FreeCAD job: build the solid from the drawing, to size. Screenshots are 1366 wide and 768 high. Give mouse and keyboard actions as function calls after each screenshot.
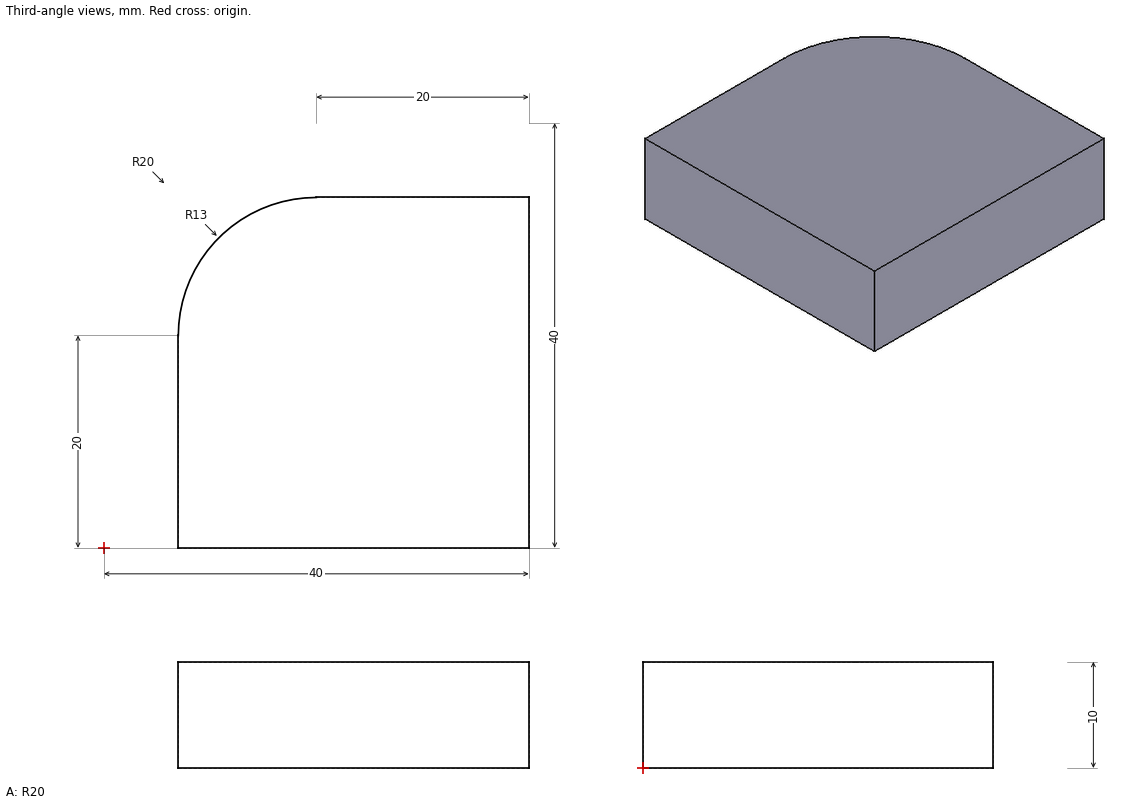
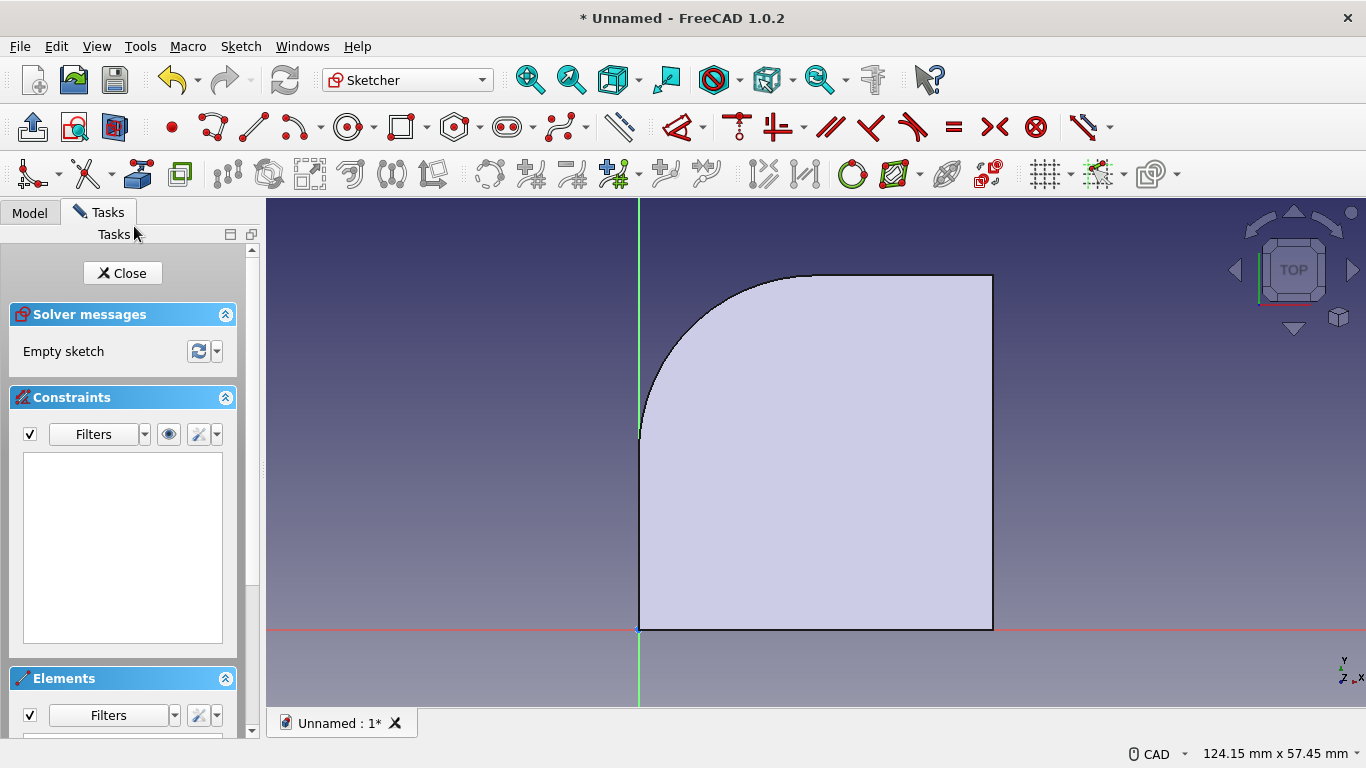
click(115, 128)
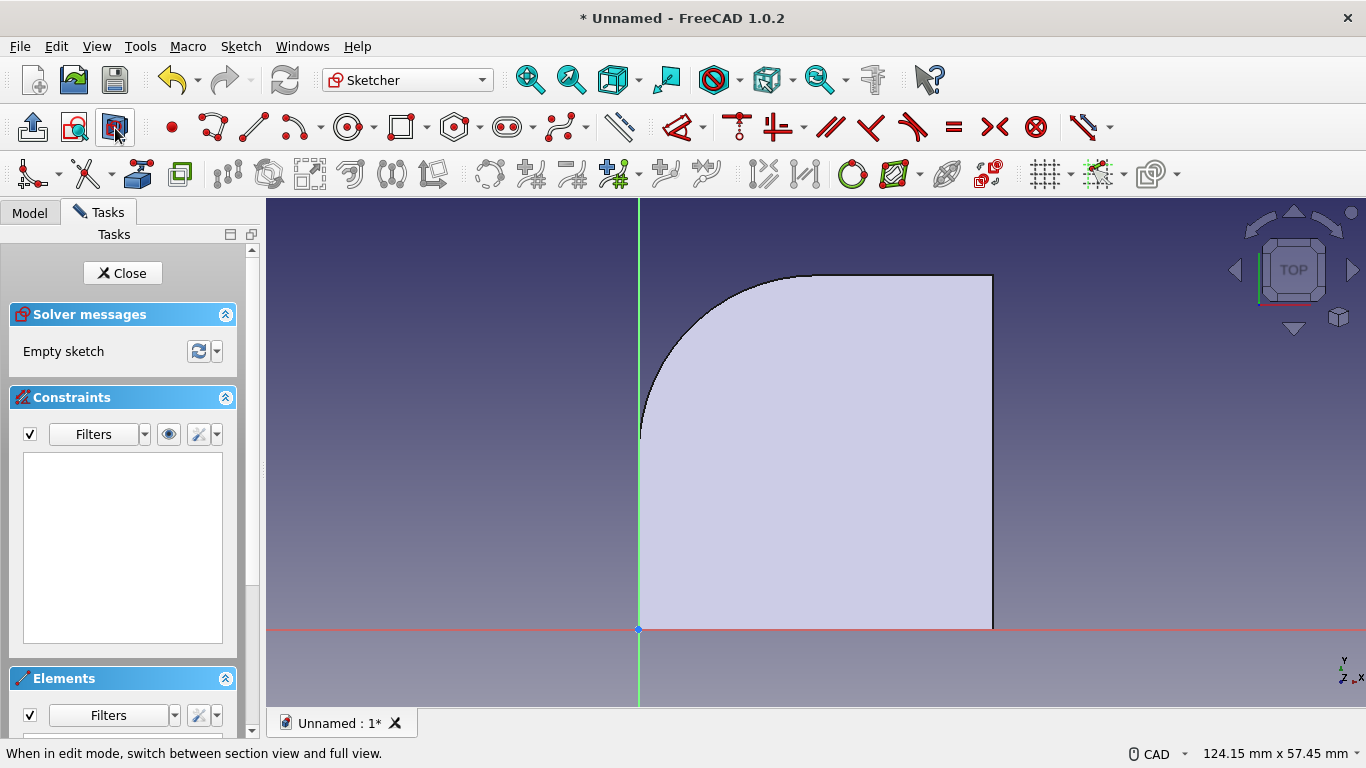
click(213, 128)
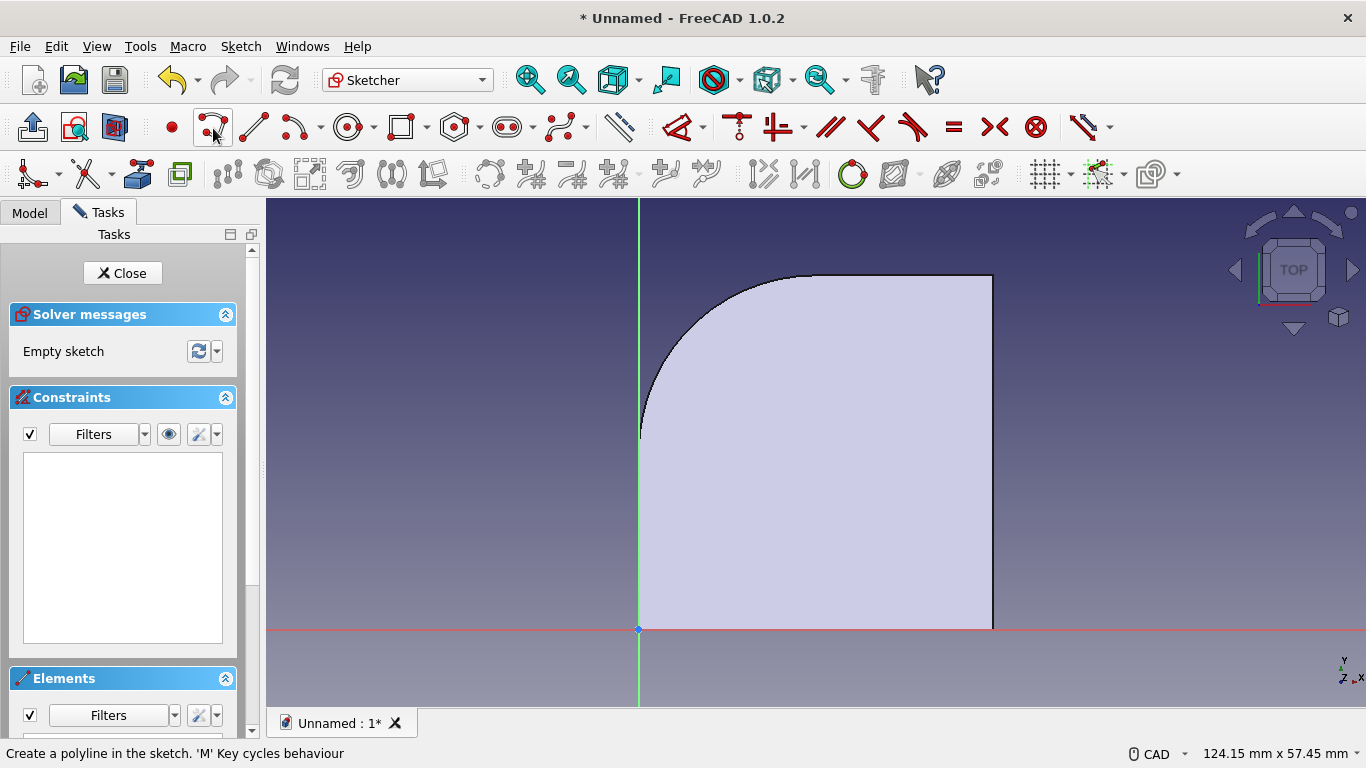
click(816, 275)
click(993, 275)
click(993, 337)
click(816, 337)
right_click(816, 337)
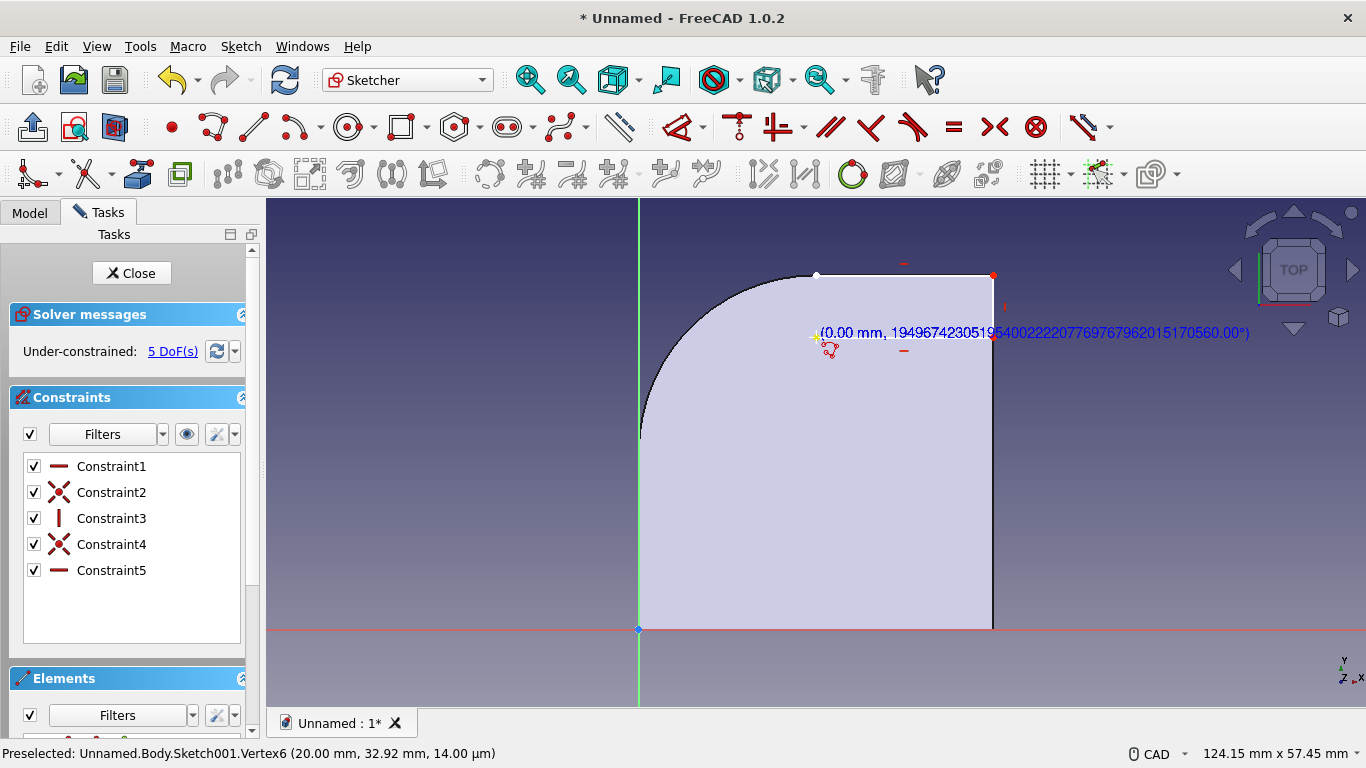
click(701, 452)
click(701, 630)
click(639, 630)
click(648, 452)
right_click(648, 452)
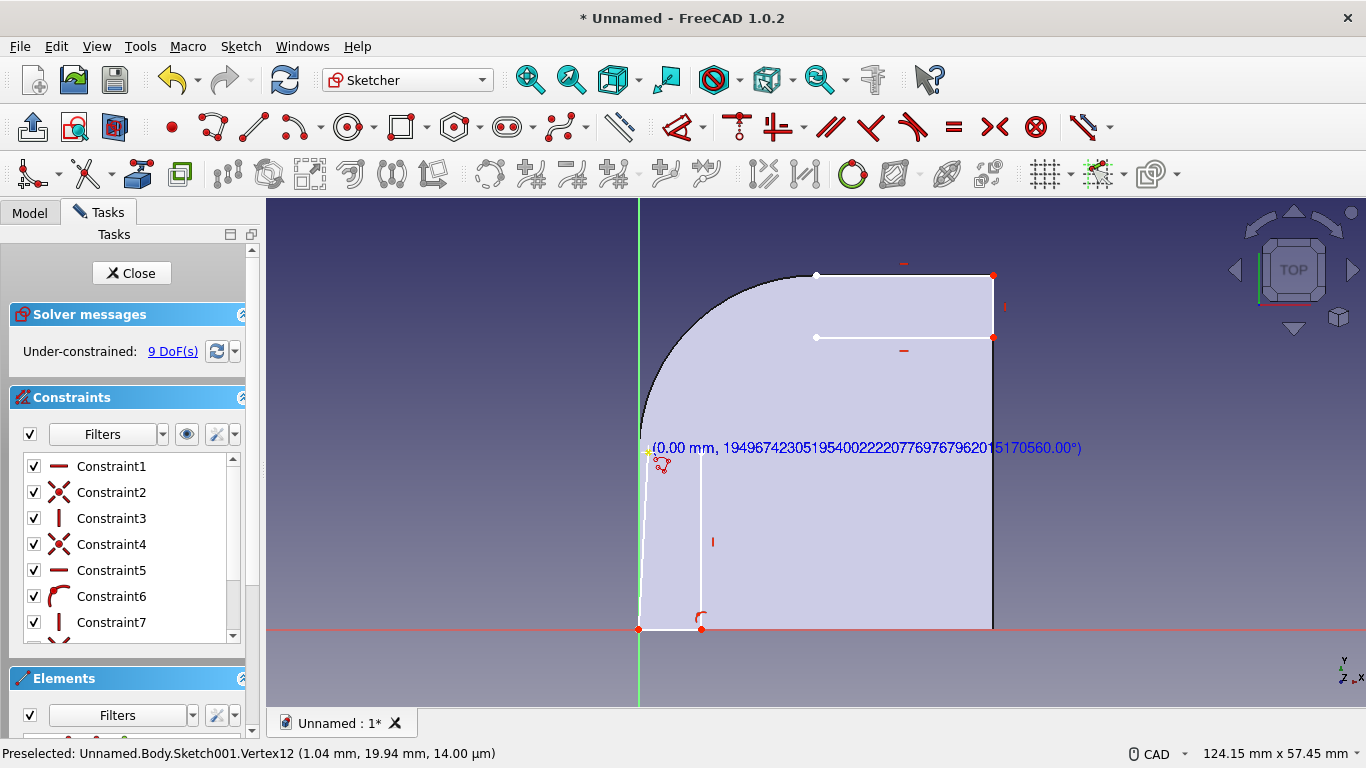
click(320, 128)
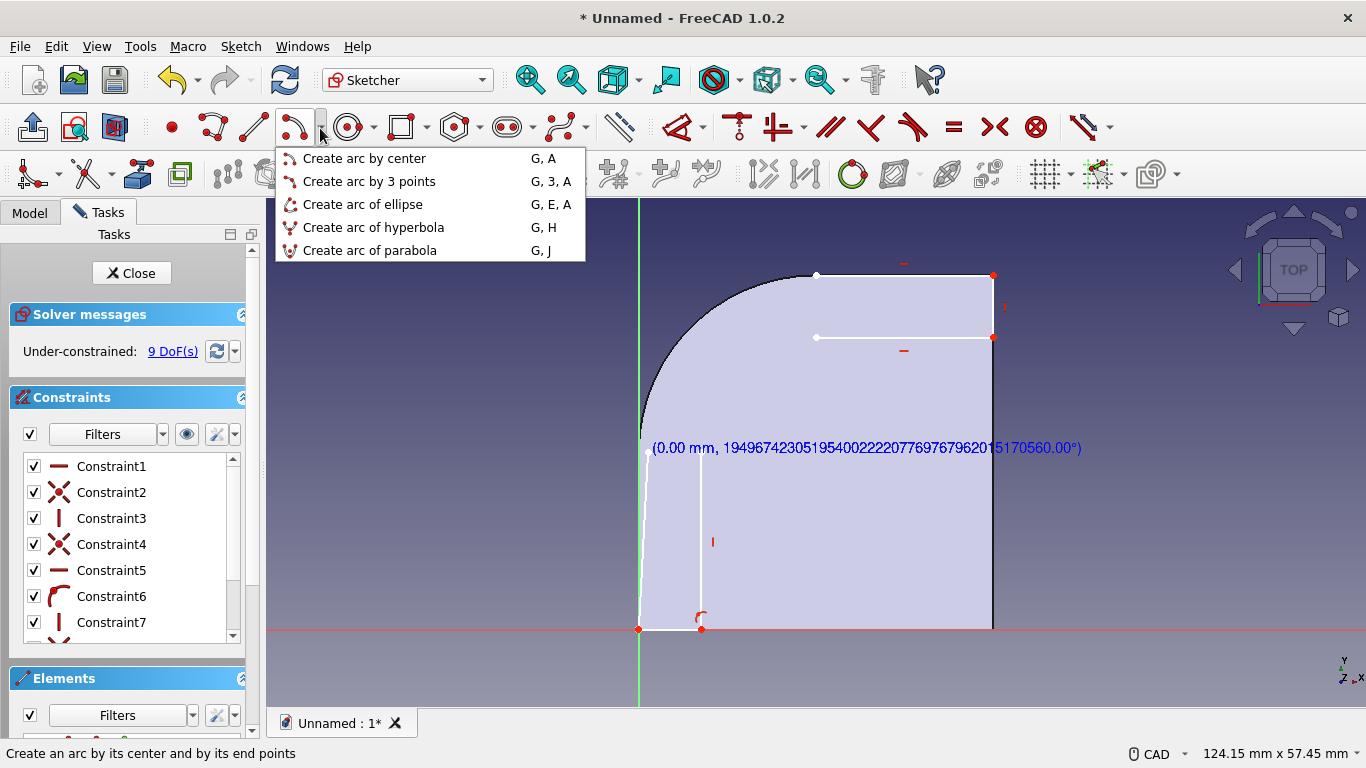
click(430, 182)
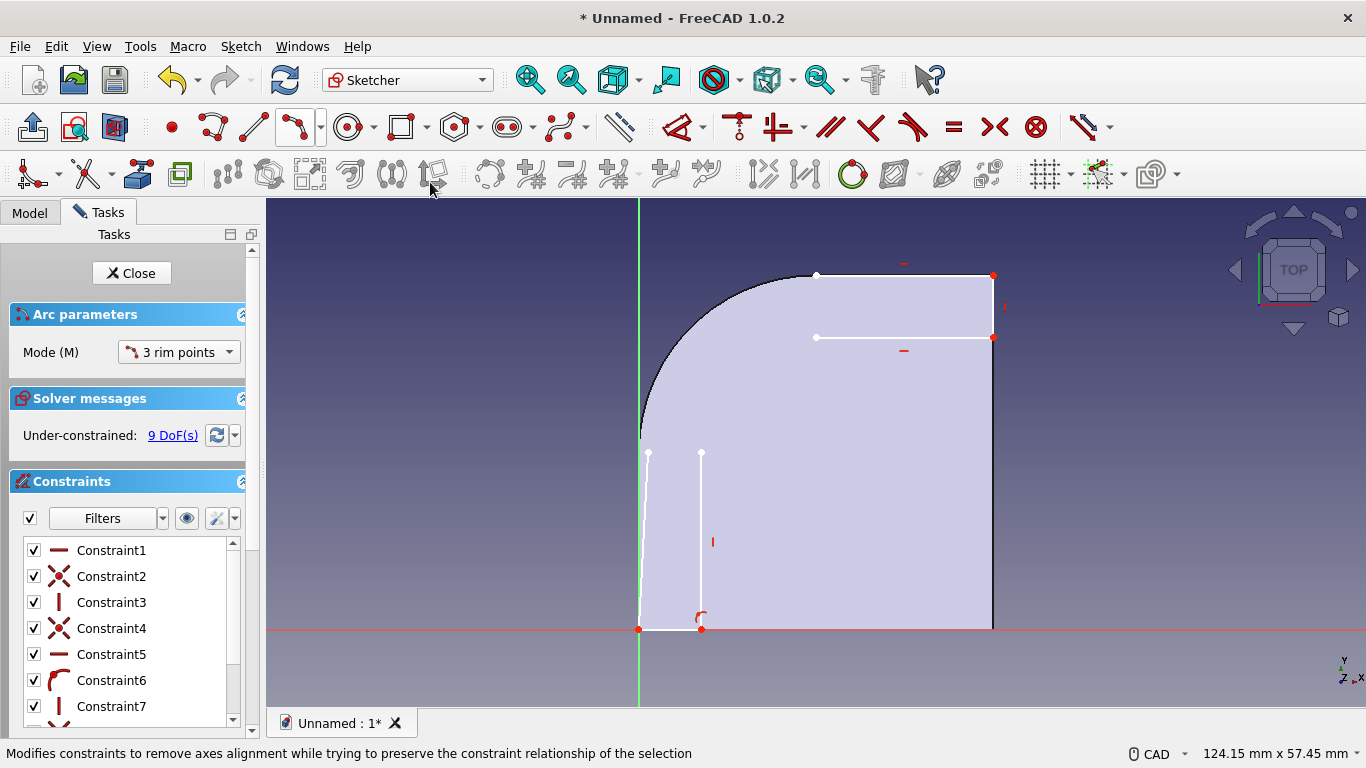
click(816, 338)
click(701, 453)
click(735, 371)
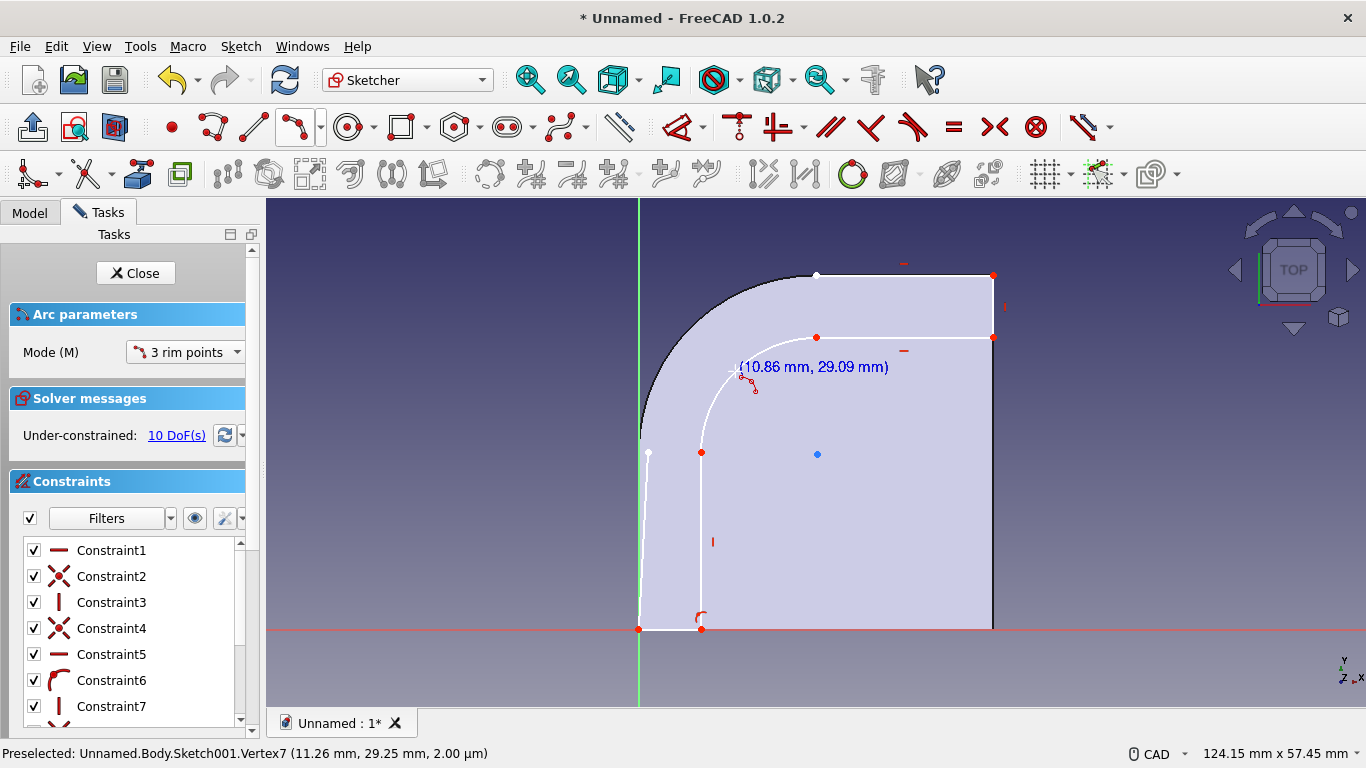
click(648, 453)
click(816, 276)
click(691, 327)
key(Escape)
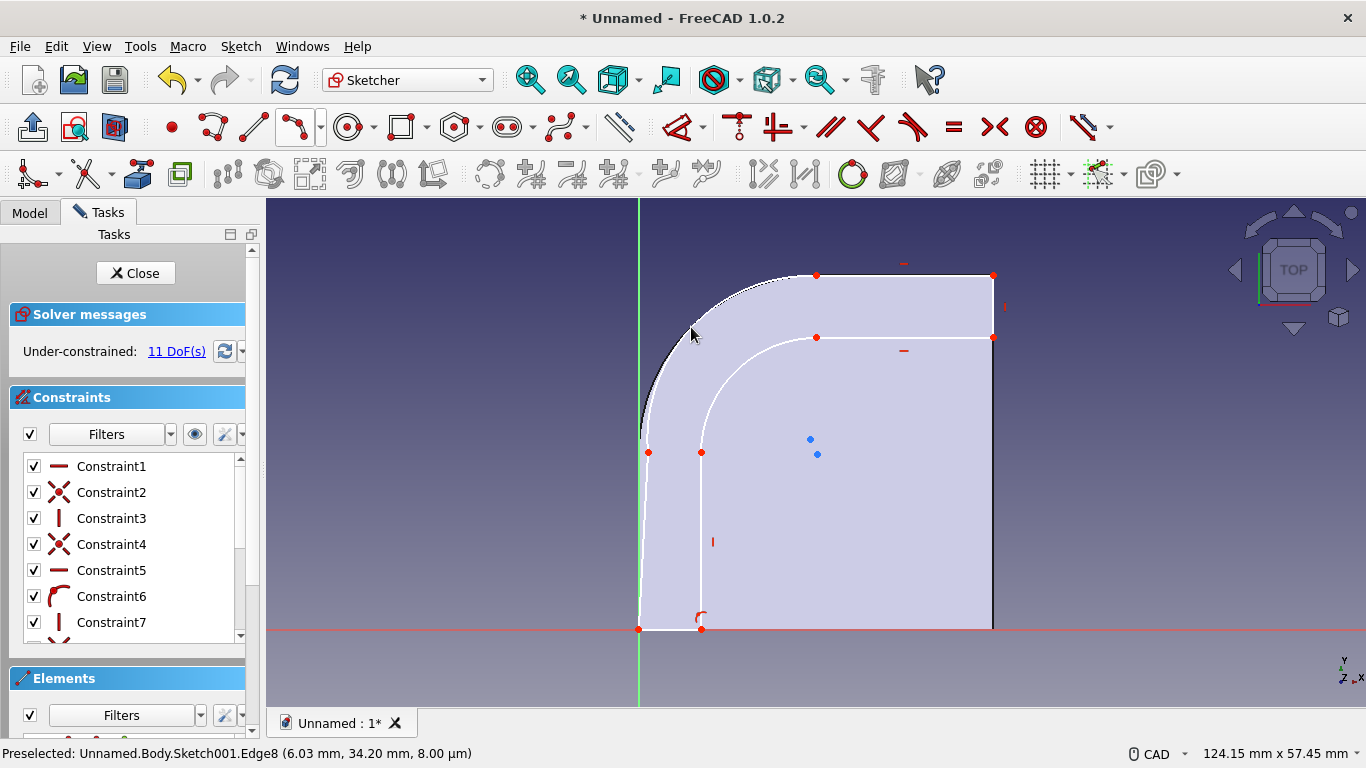
click(869, 276)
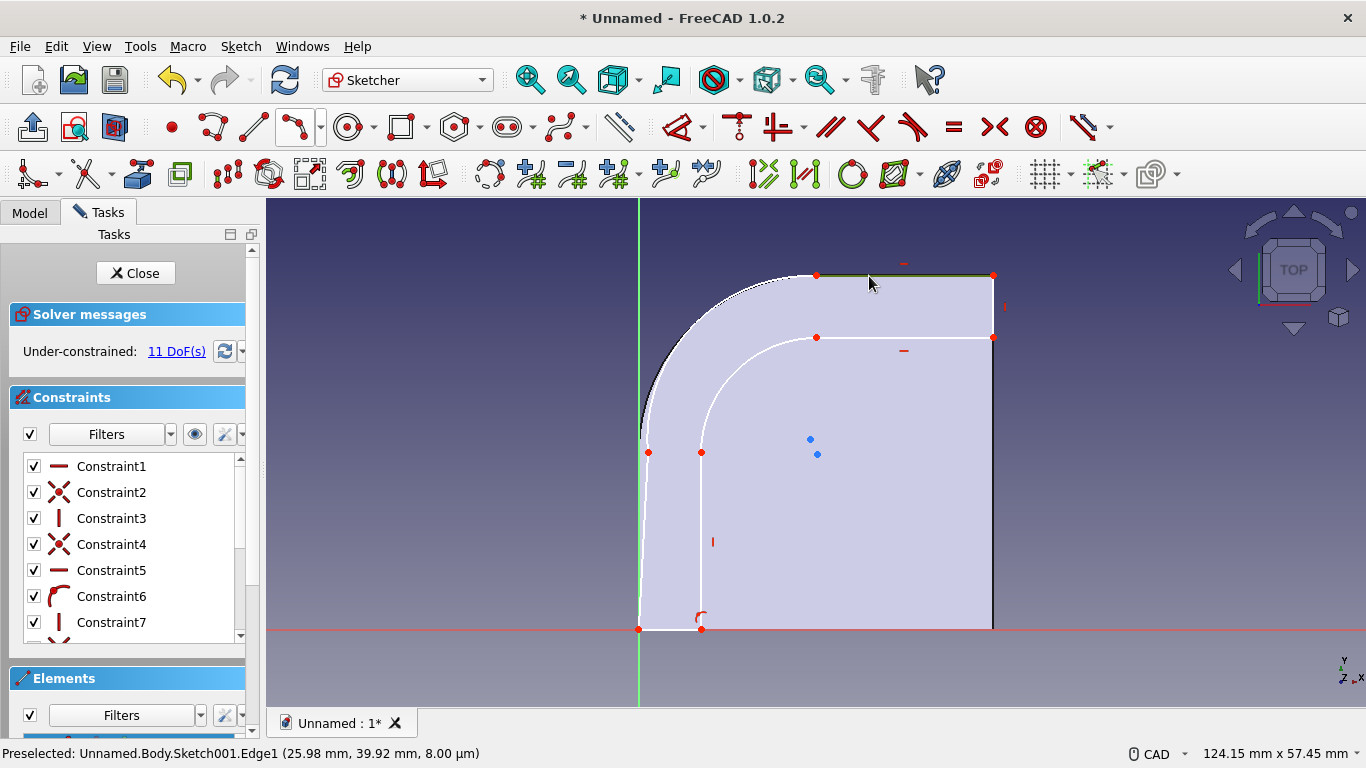
click(736, 294)